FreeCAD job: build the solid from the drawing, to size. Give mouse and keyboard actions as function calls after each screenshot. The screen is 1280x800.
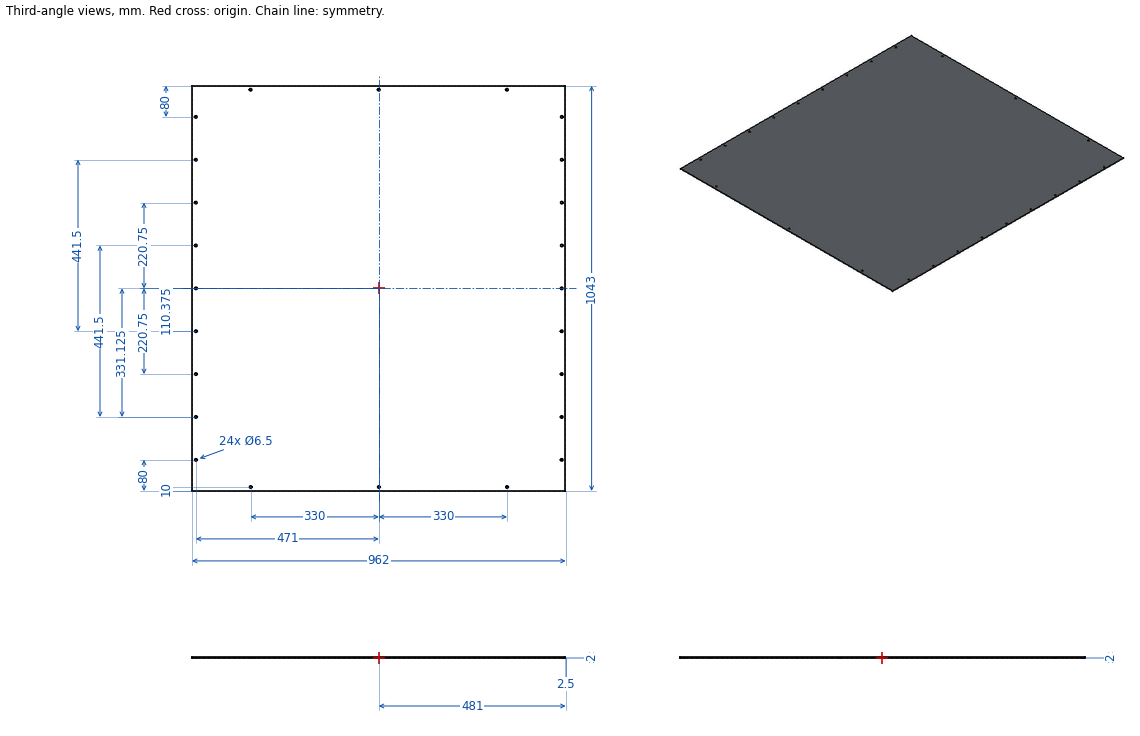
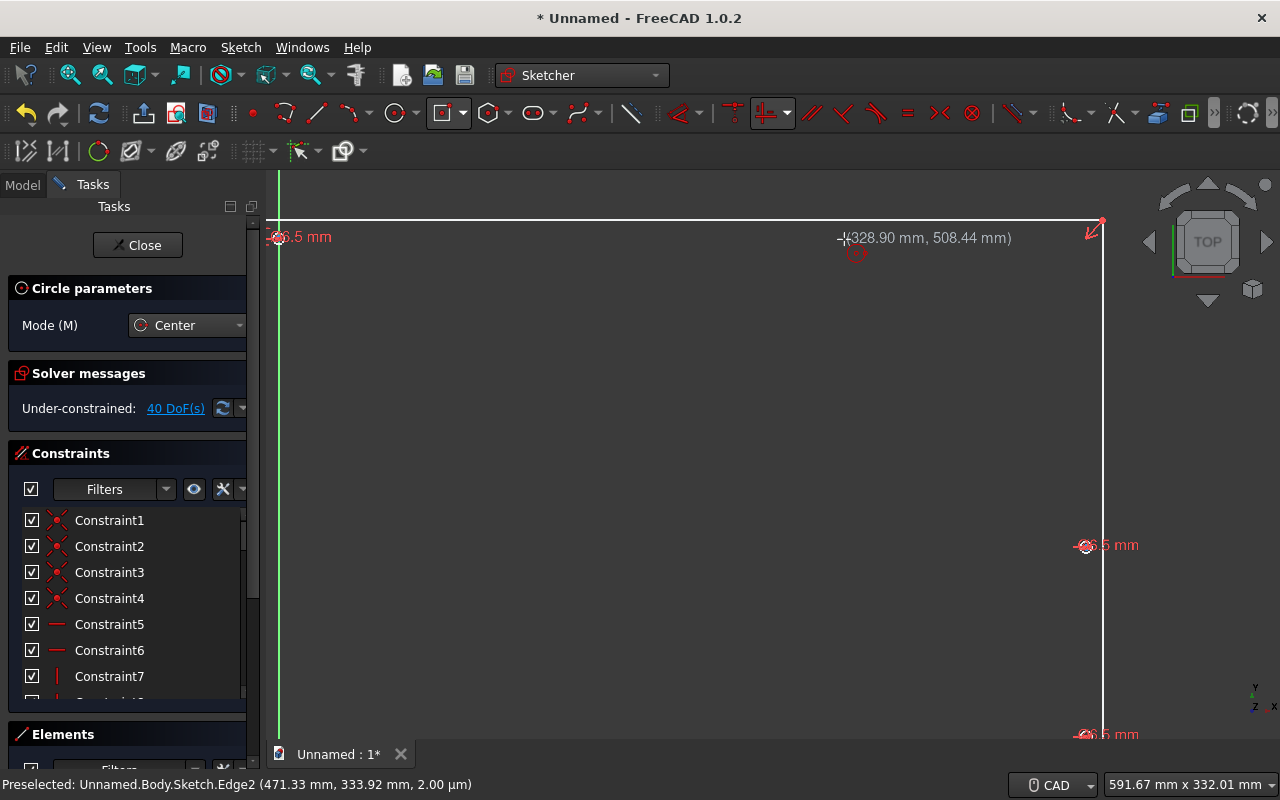
click(844, 237)
move(848, 241)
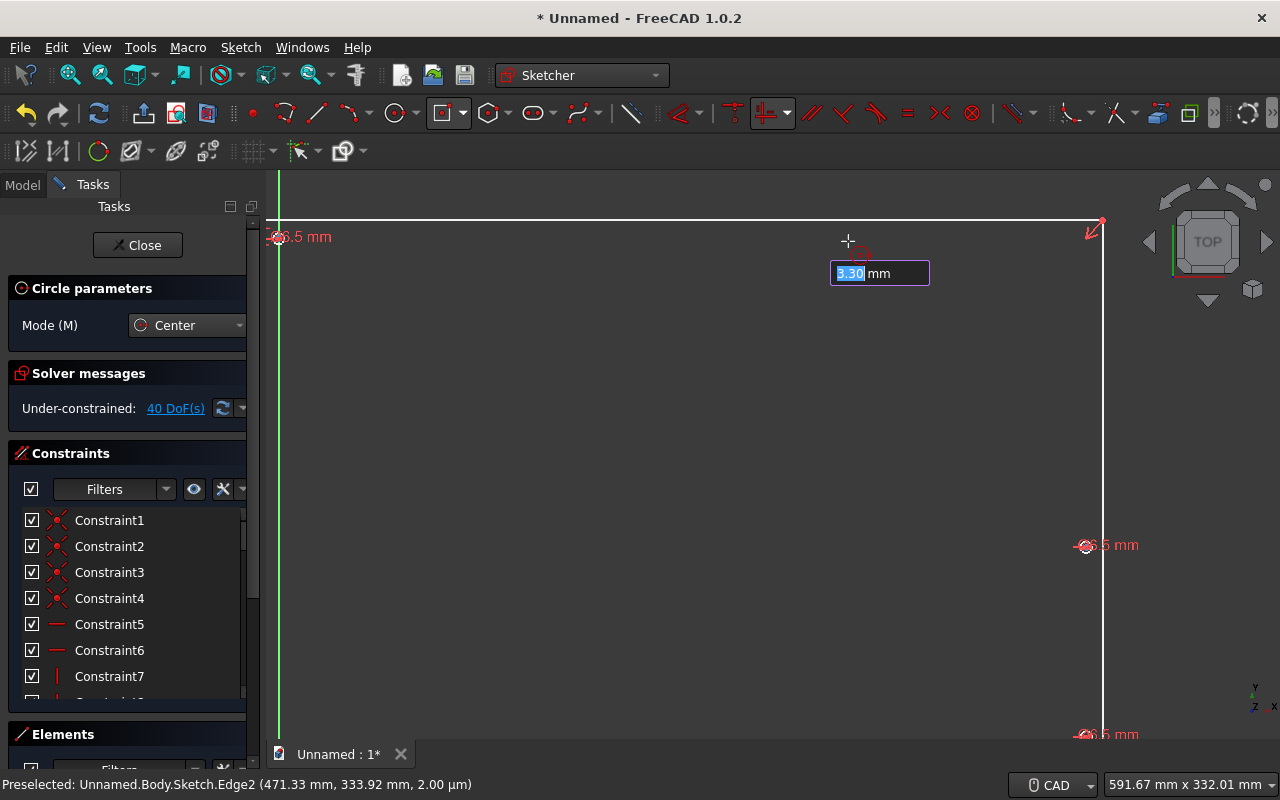
text(6.5)
key(Return)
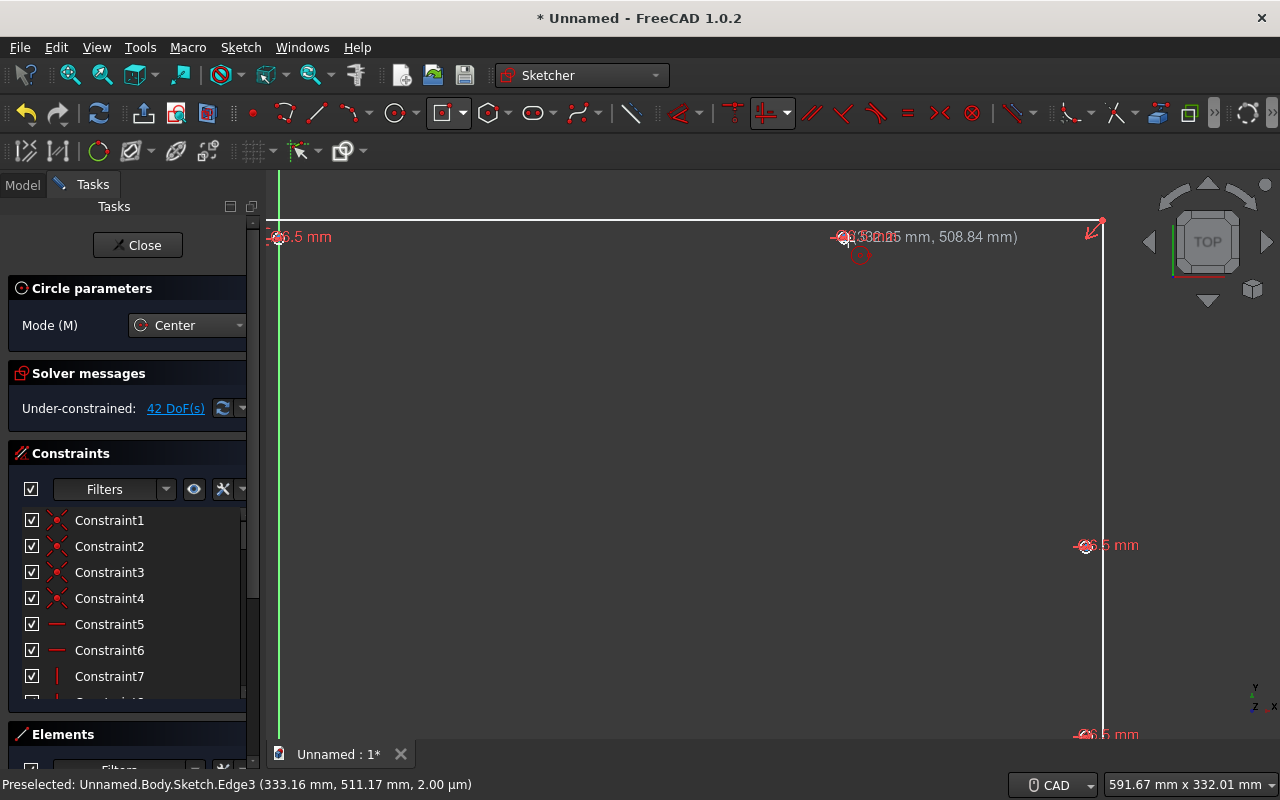
scroll(1086, 357, up, 8)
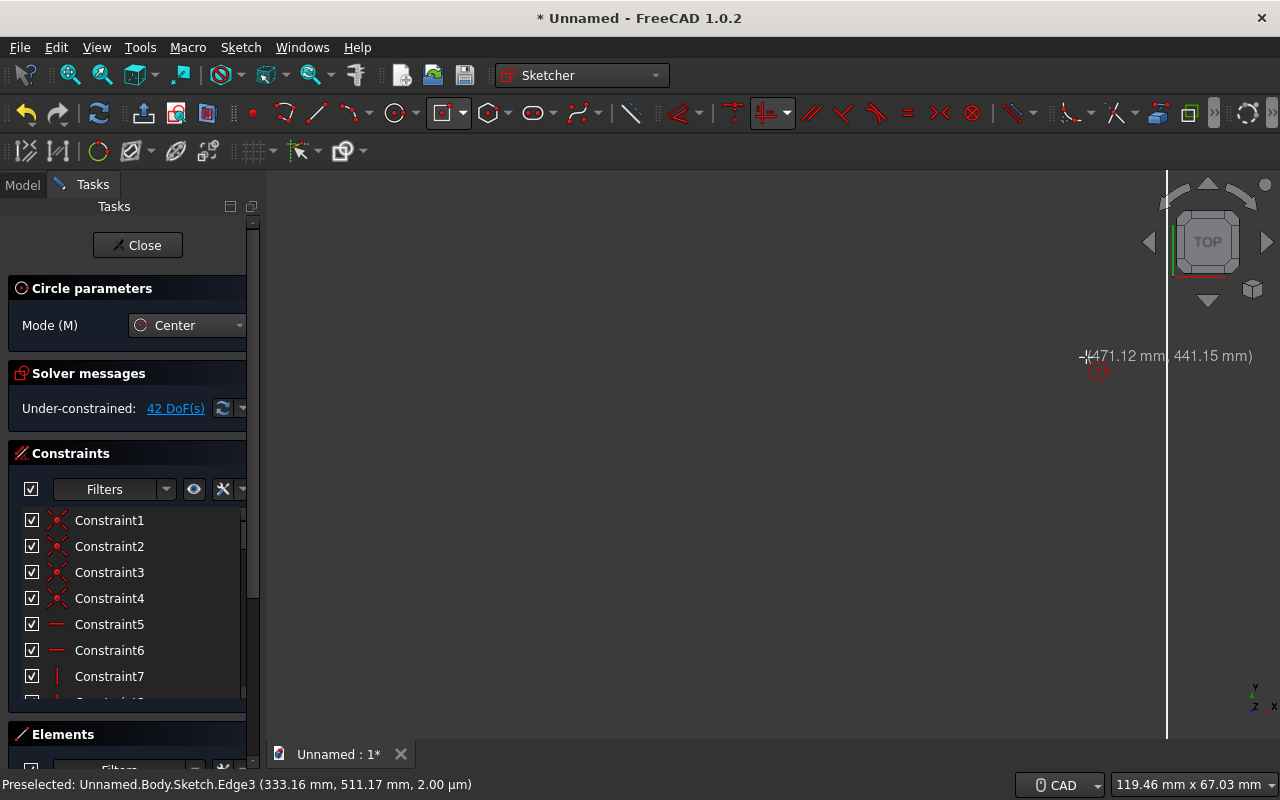
scroll(894, 263, down, 15)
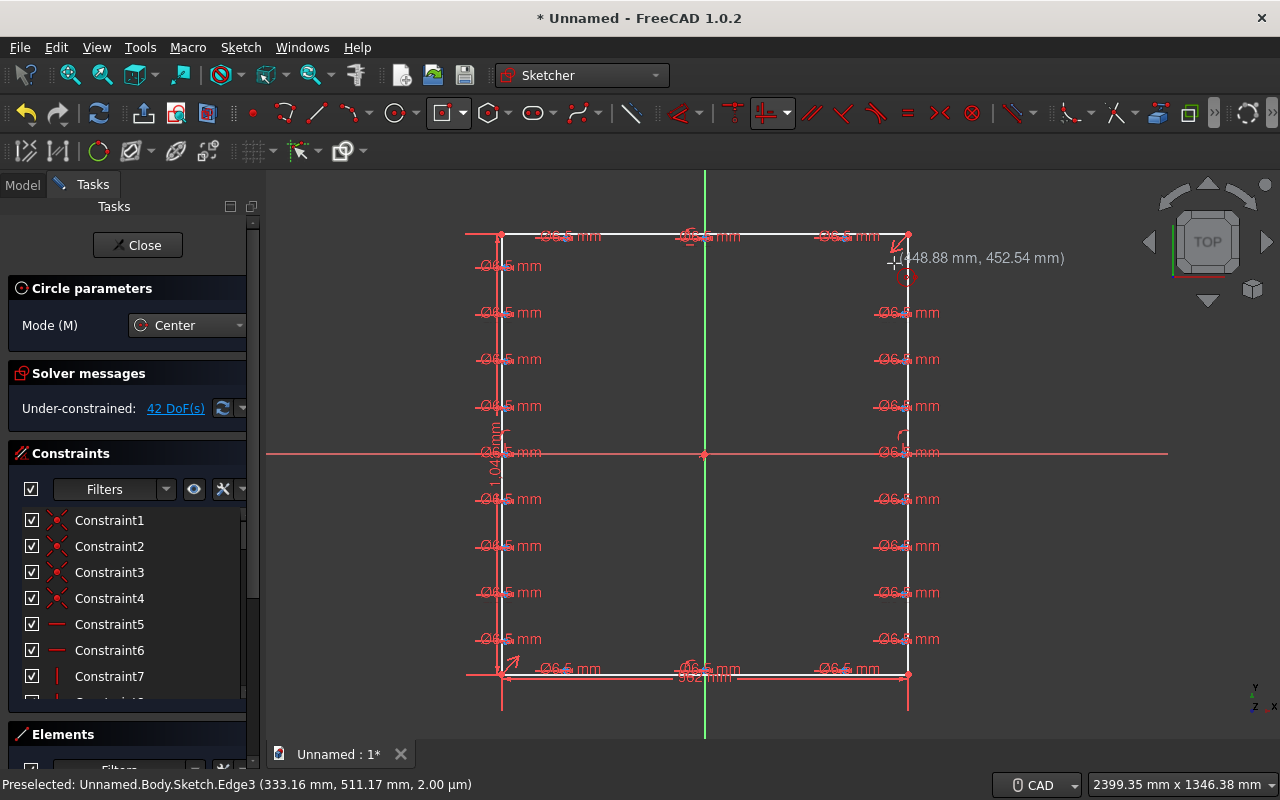
scroll(904, 268, up, 7)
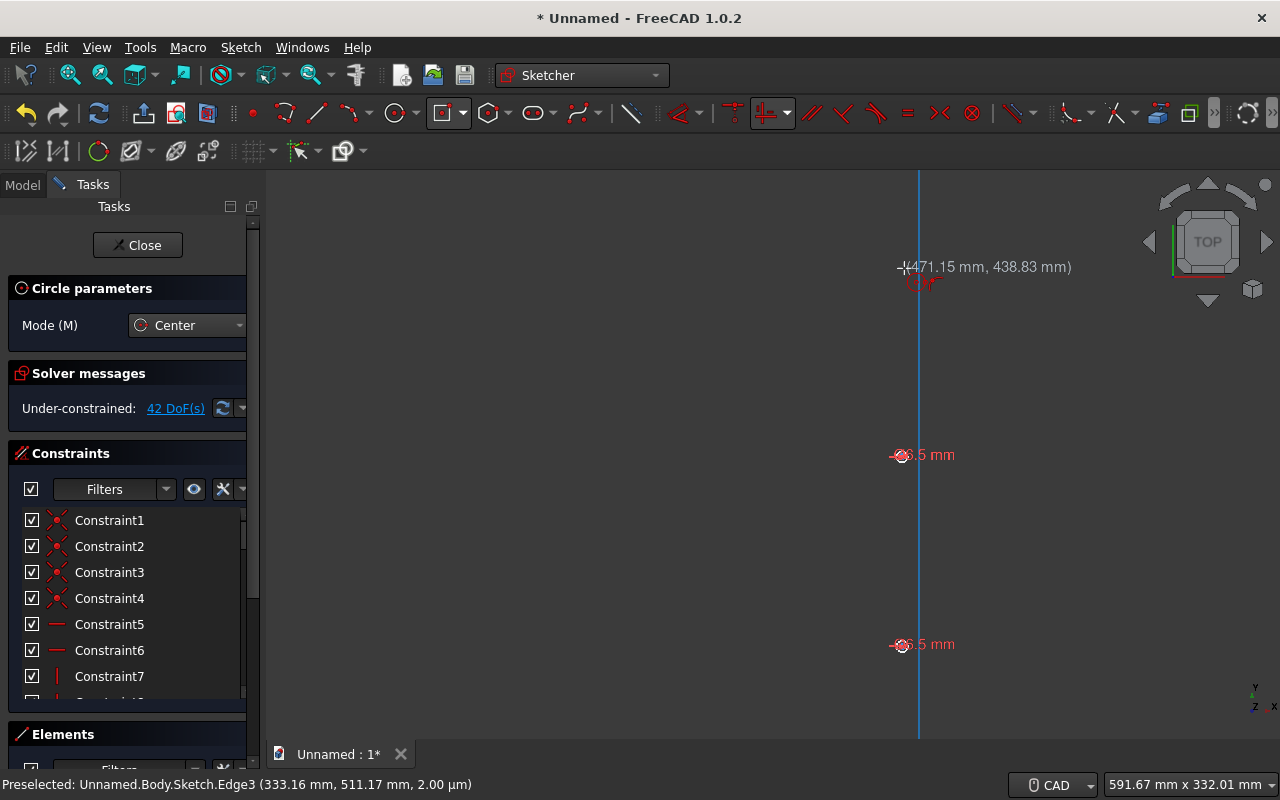
click(902, 267)
move(898, 263)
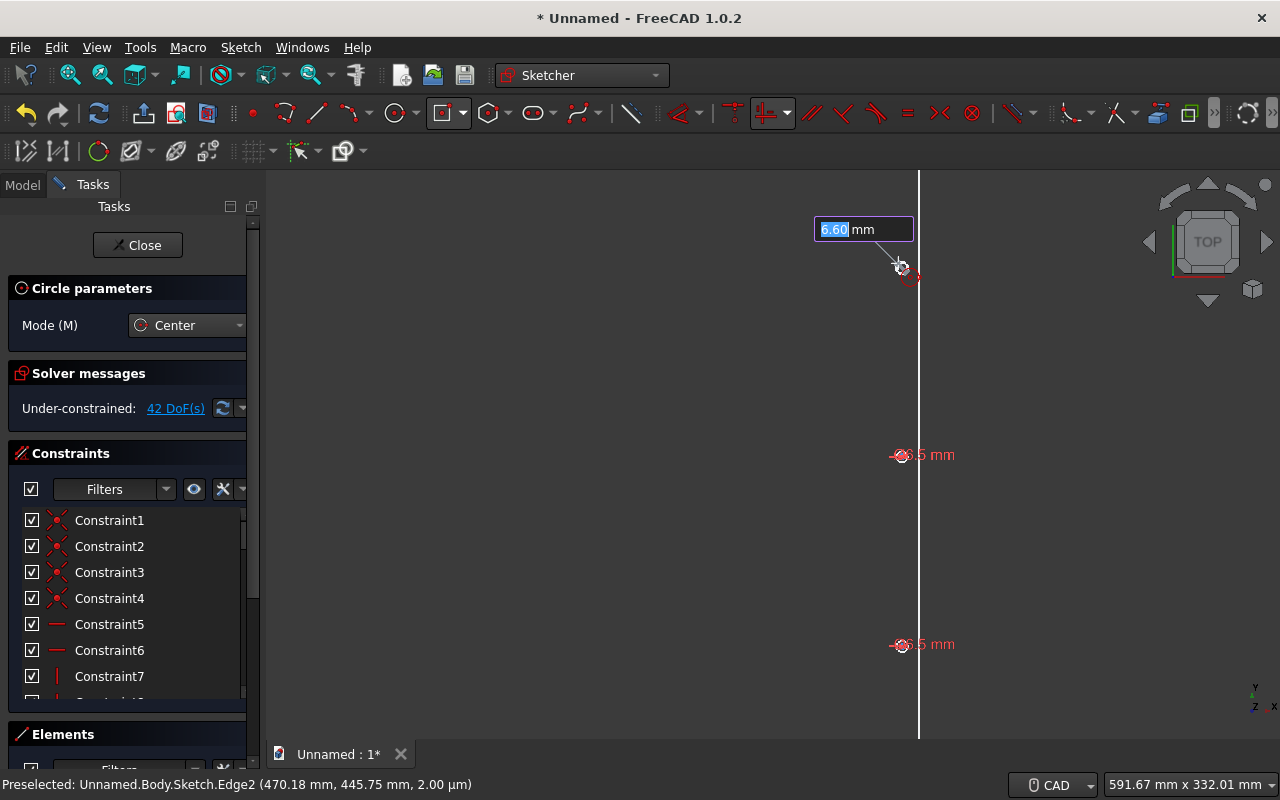
text(6.5)
key(Return)
key(Escape)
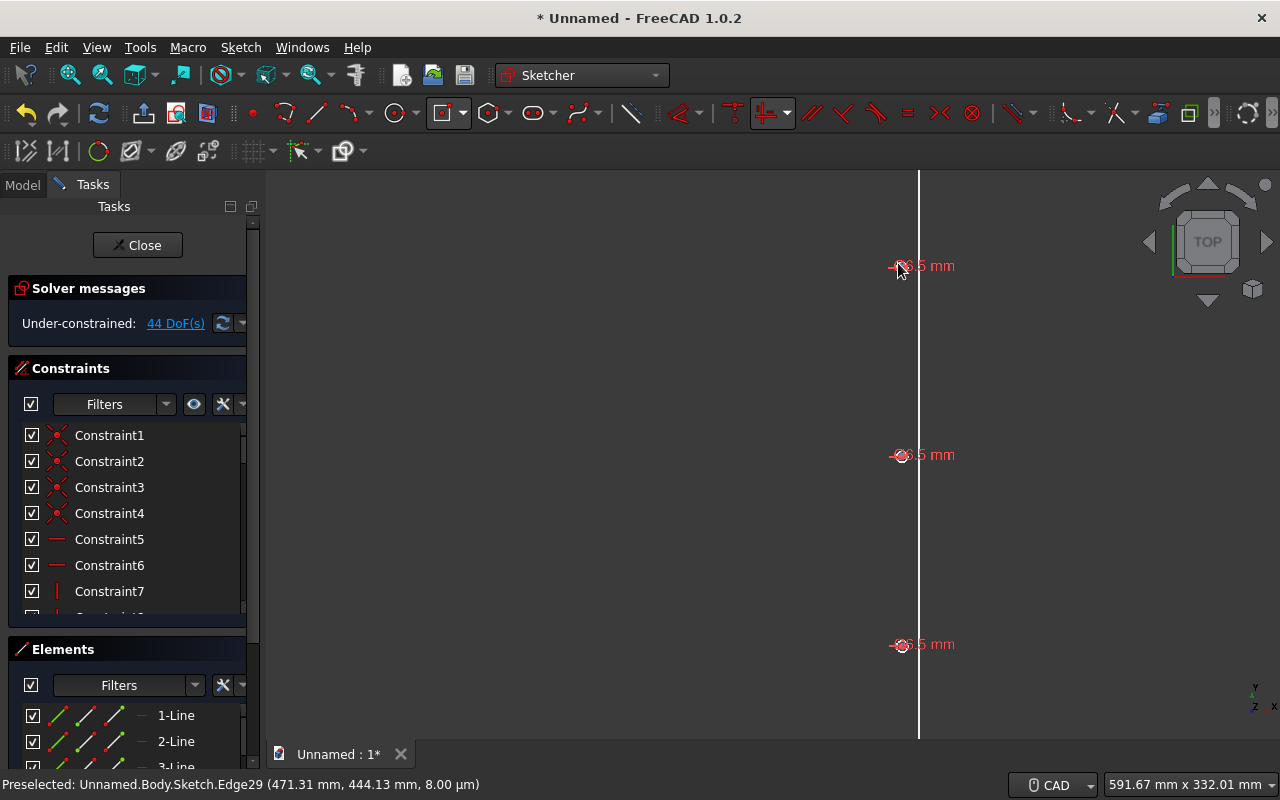
scroll(859, 311, down, 8)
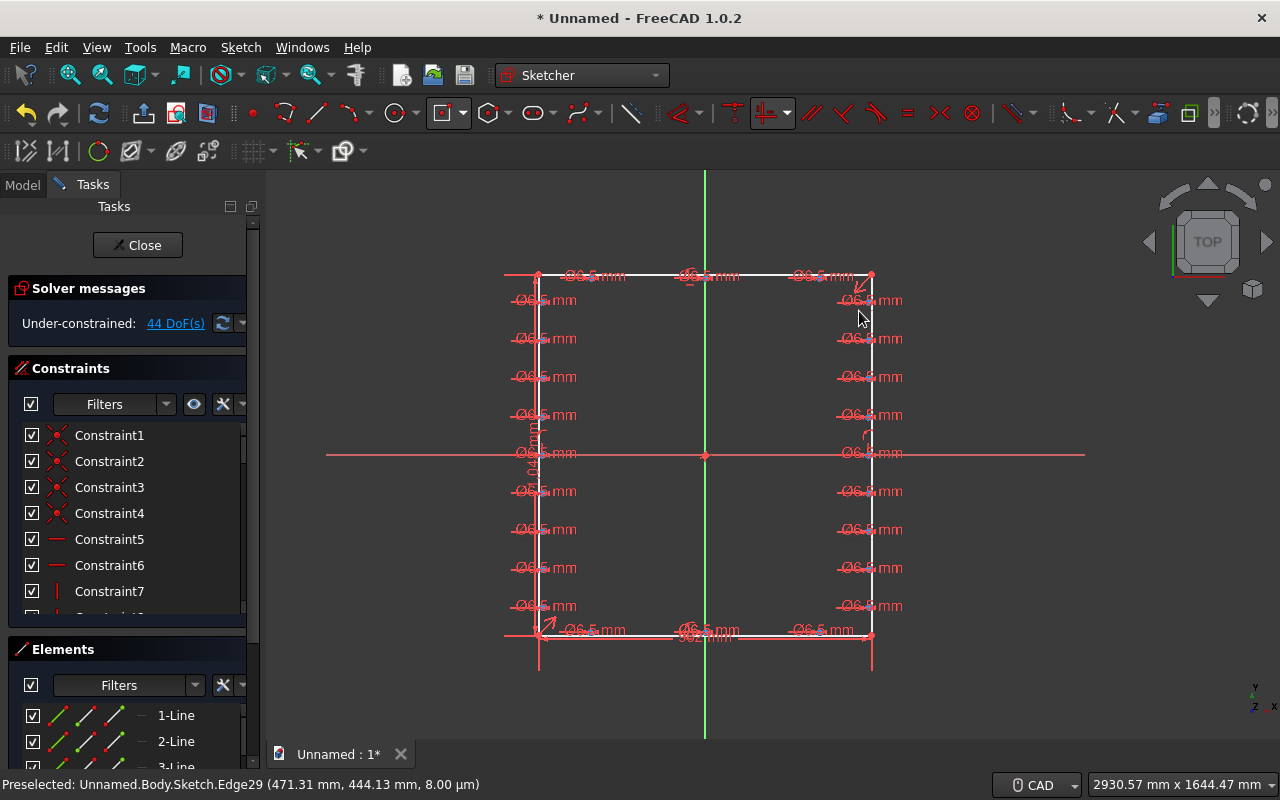
click(542, 608)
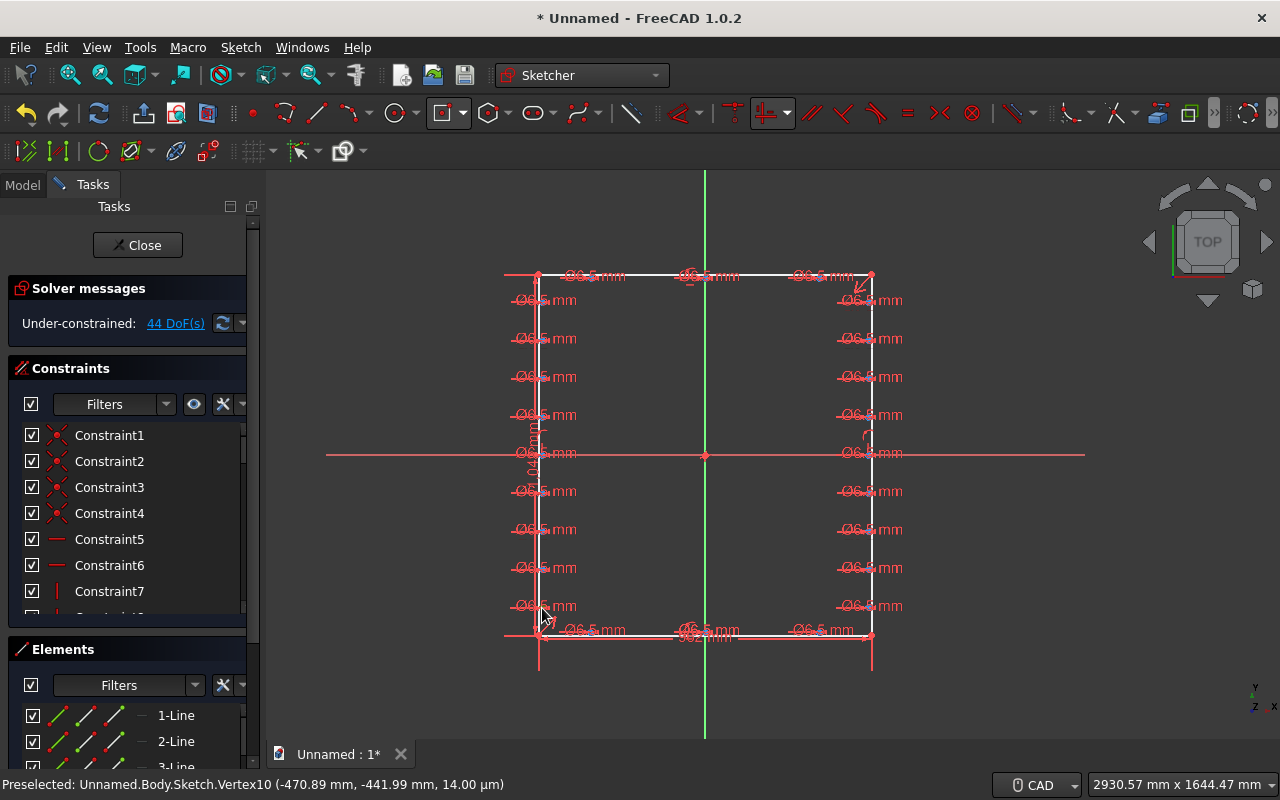
click(542, 570)